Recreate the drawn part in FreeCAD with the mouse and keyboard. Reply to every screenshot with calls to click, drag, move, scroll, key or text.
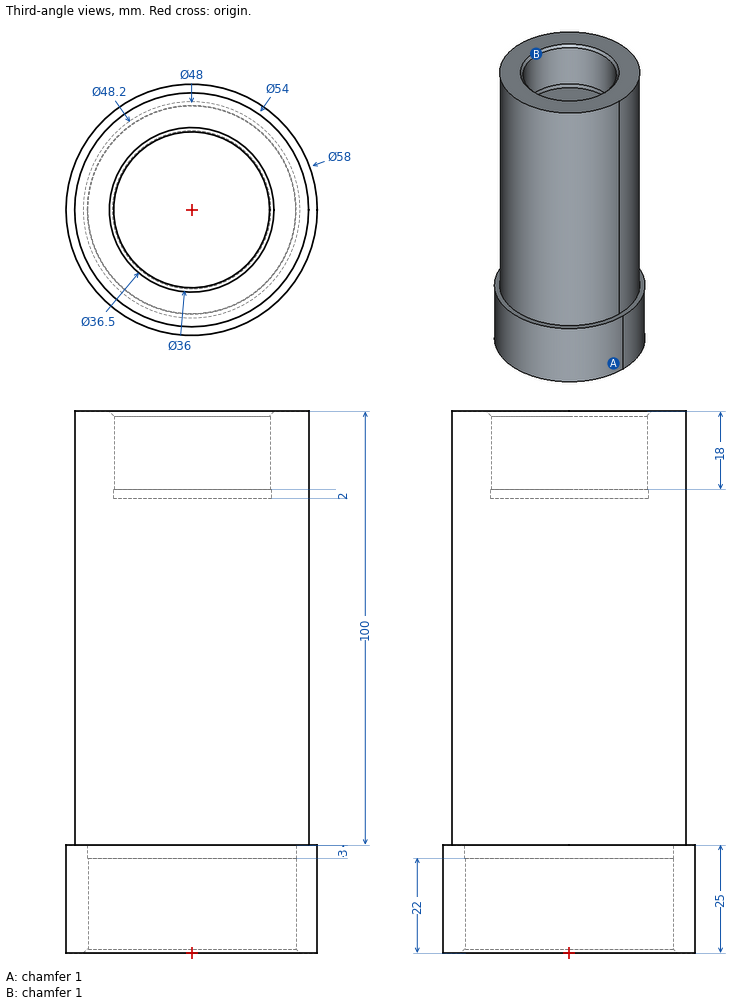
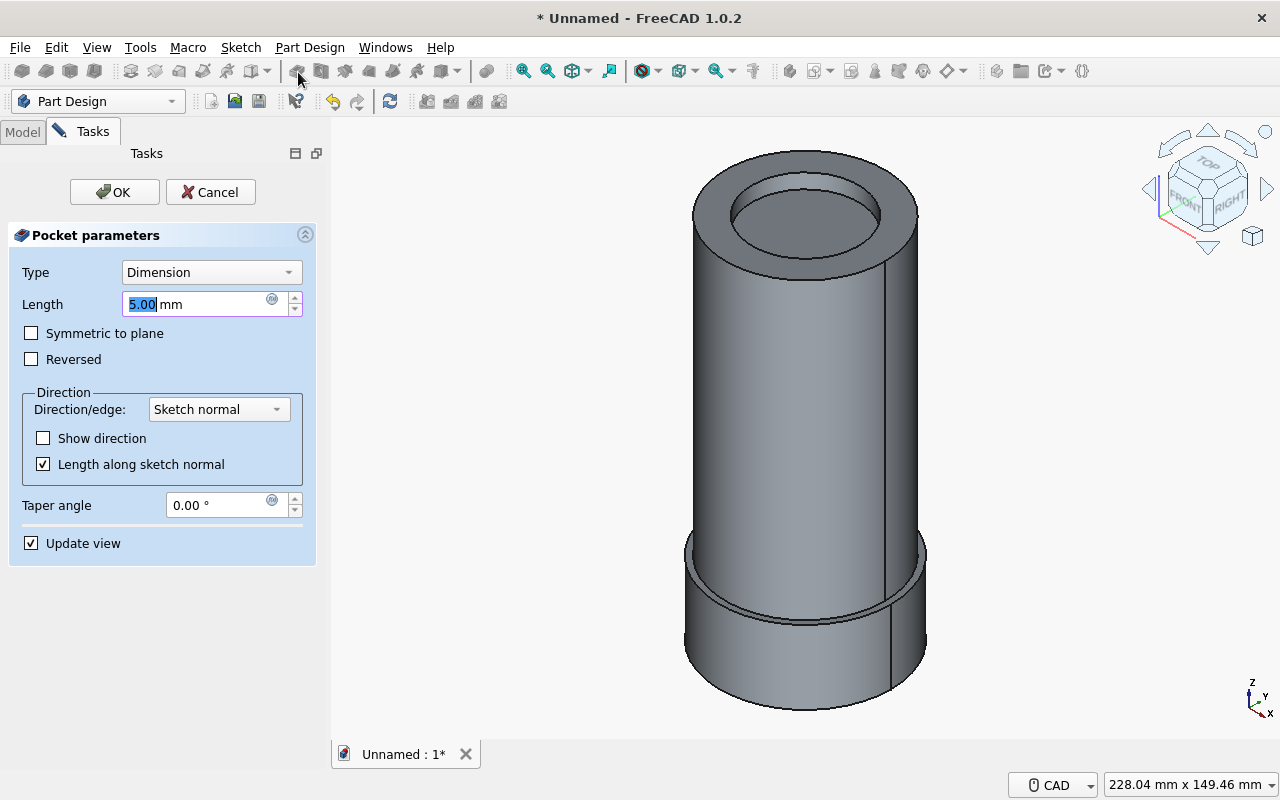
text(18)
key(Tab)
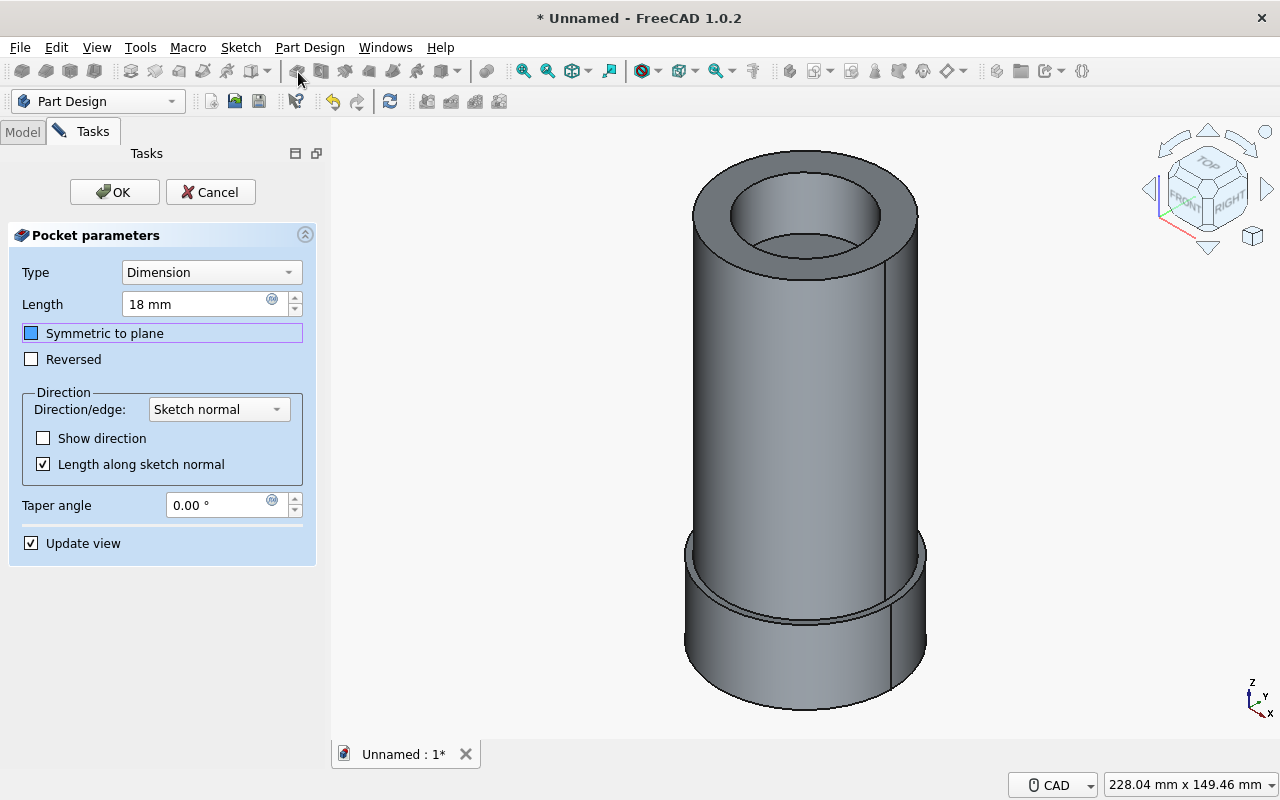
click(115, 192)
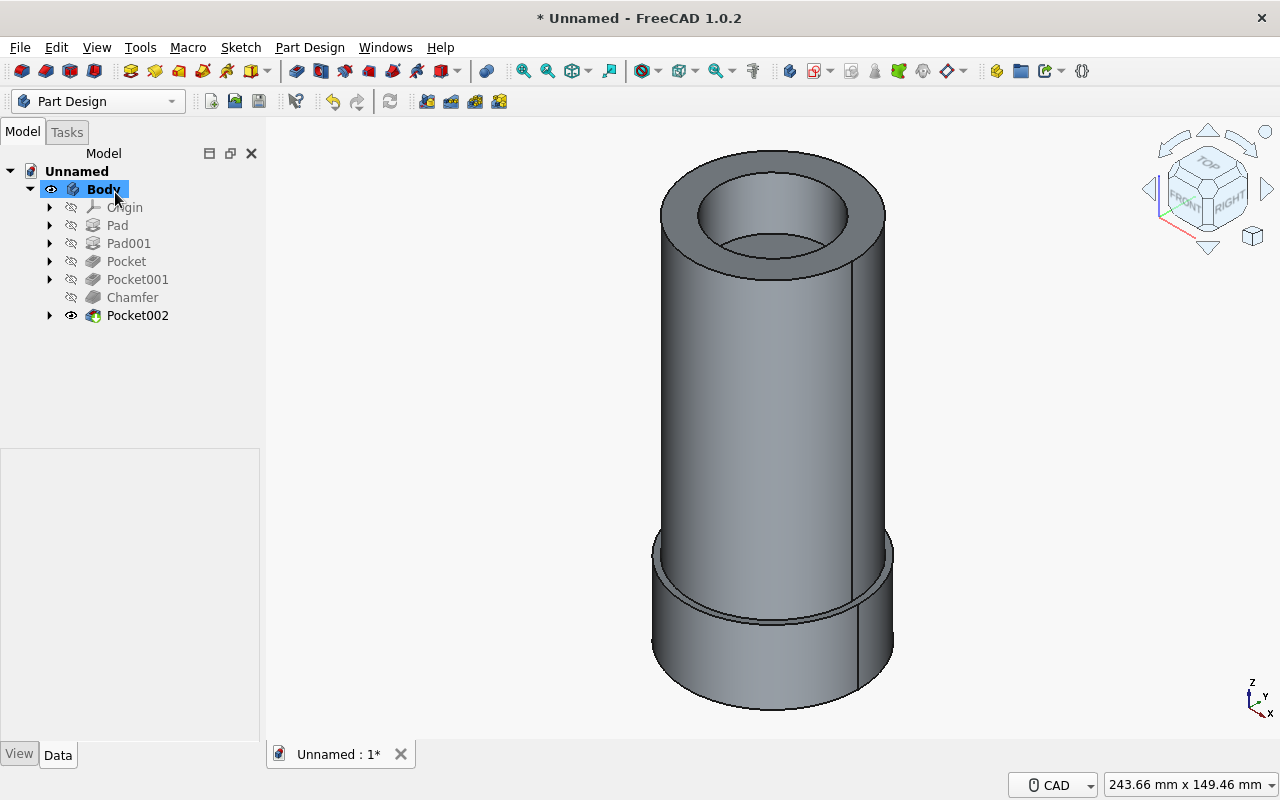
click(524, 72)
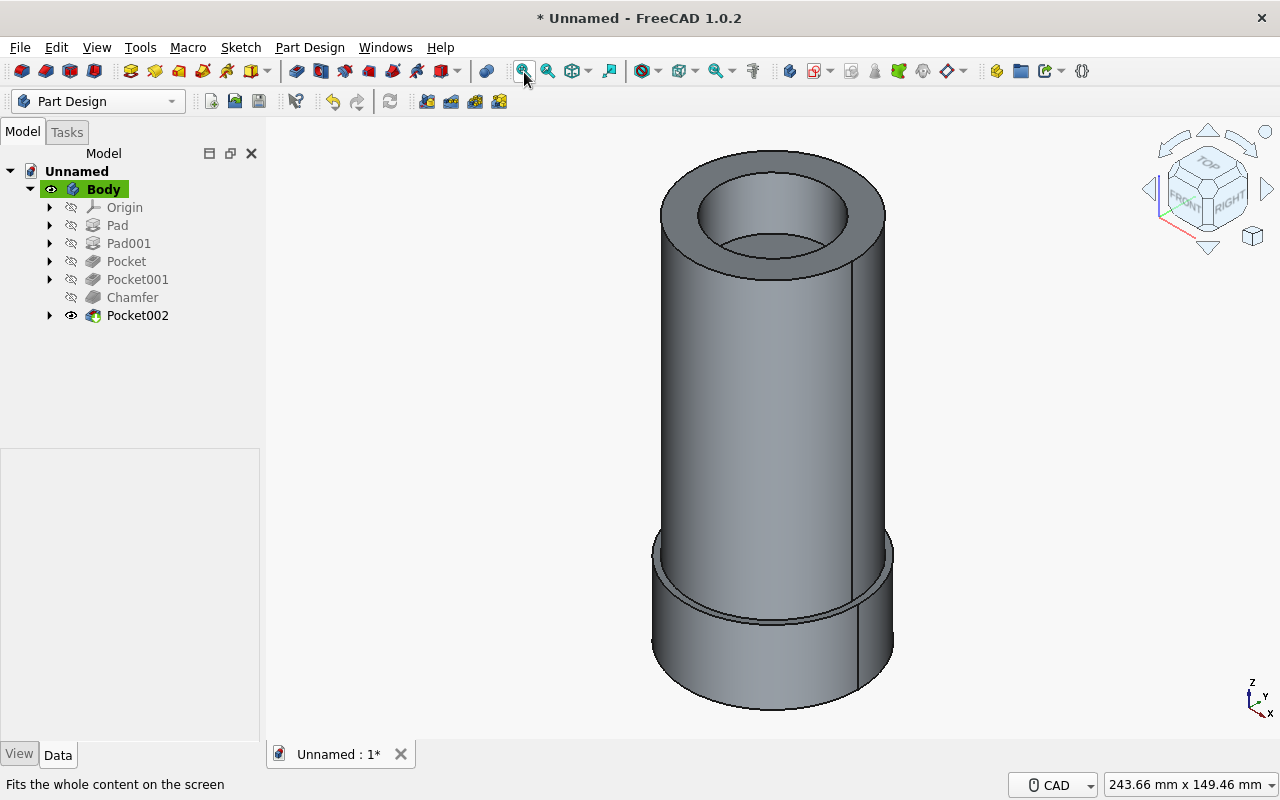
key(2)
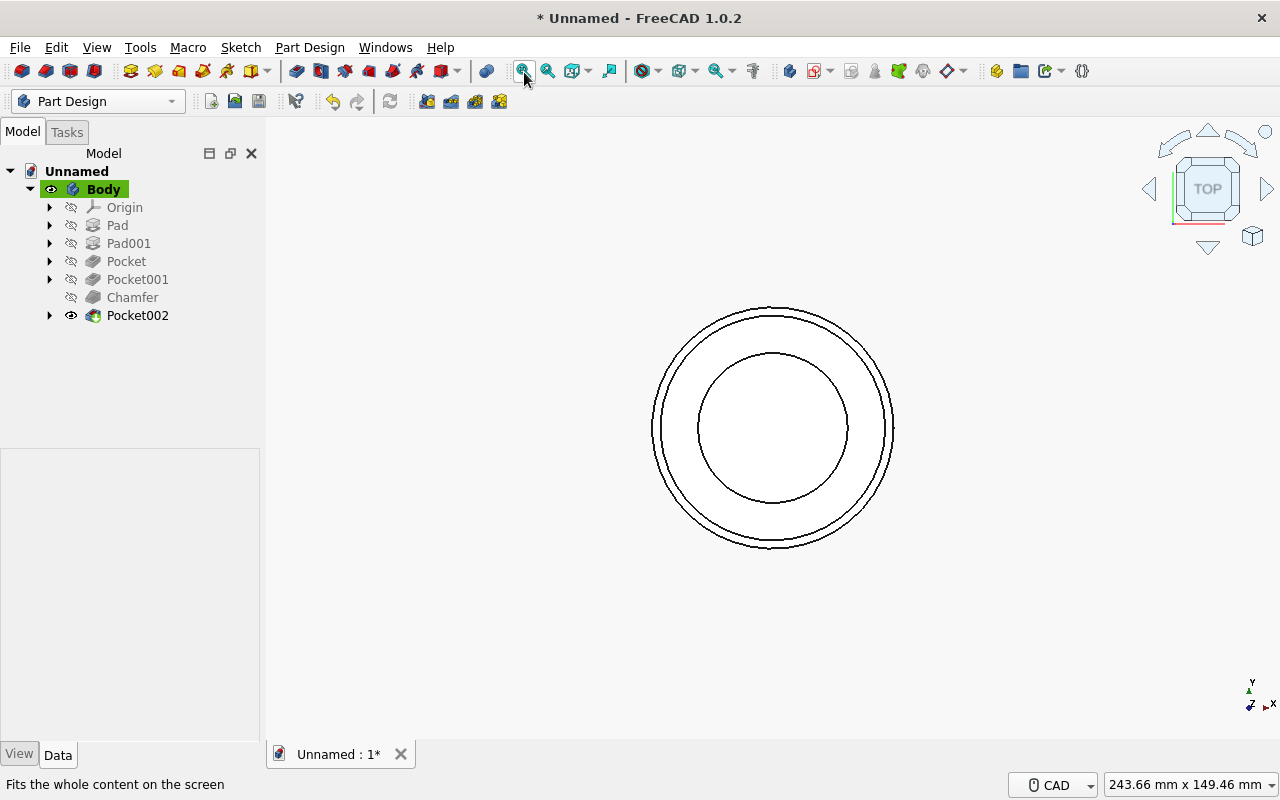
click(524, 72)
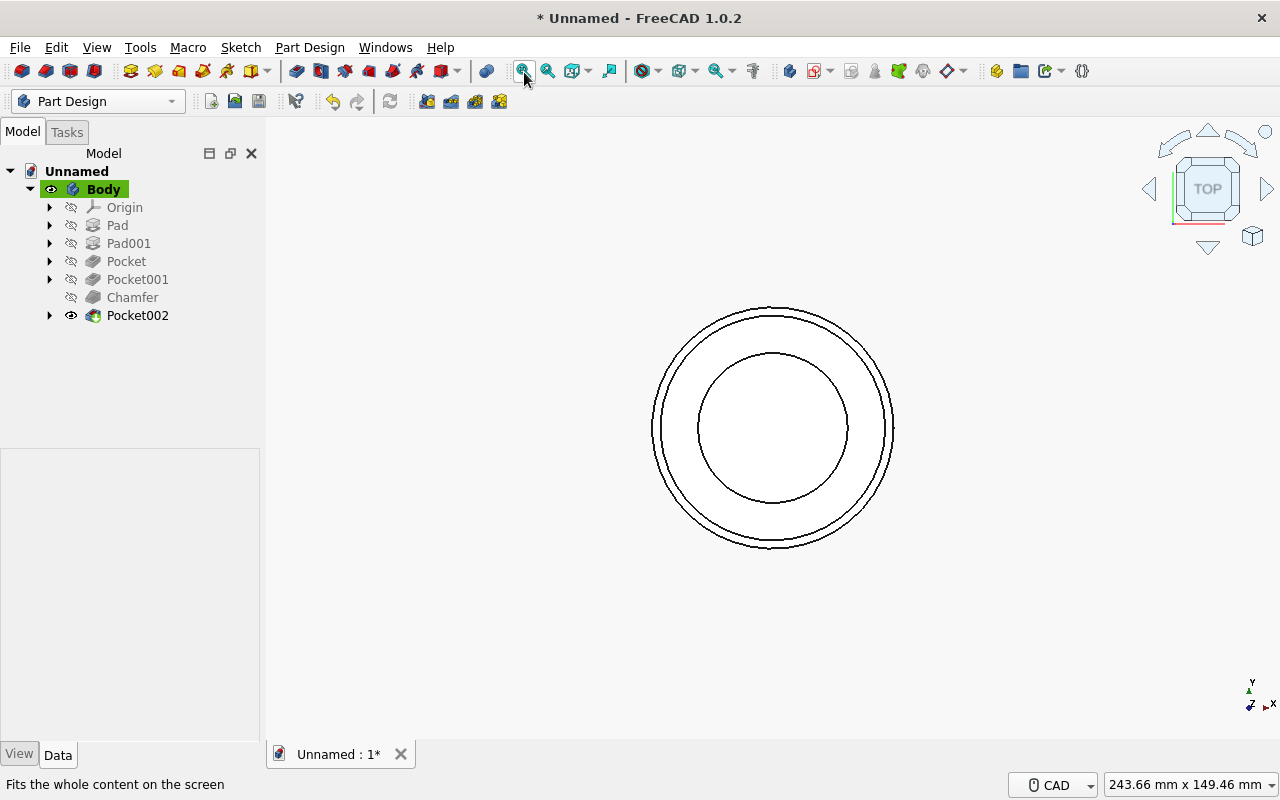
click(773, 427)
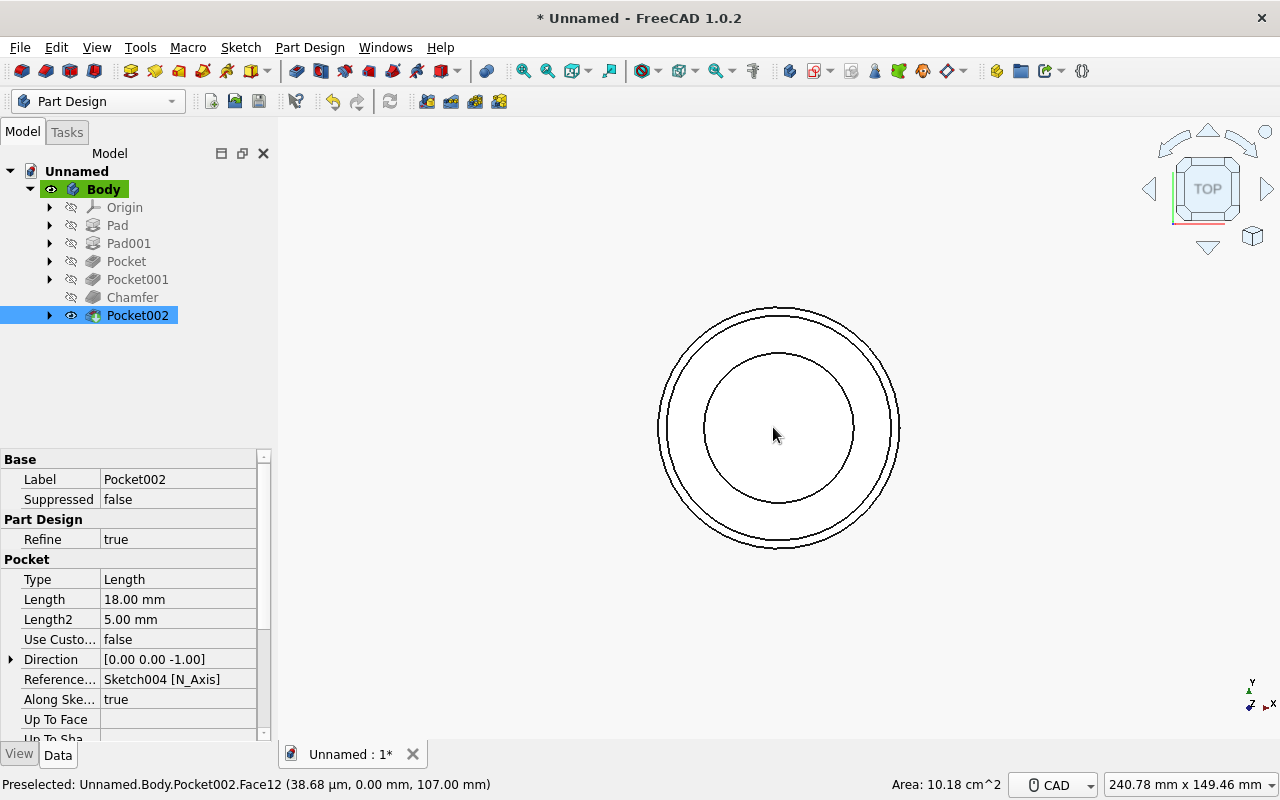
click(814, 72)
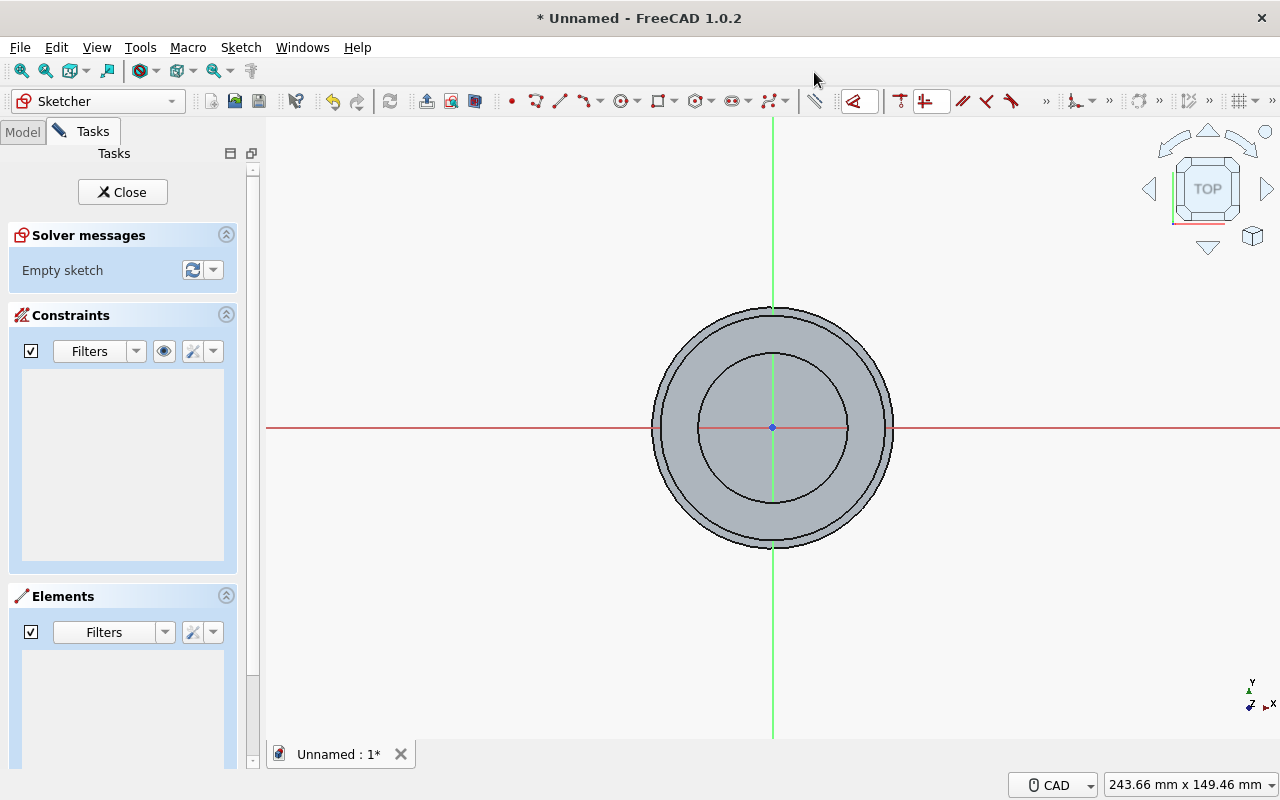
scroll(813, 428, up, 5)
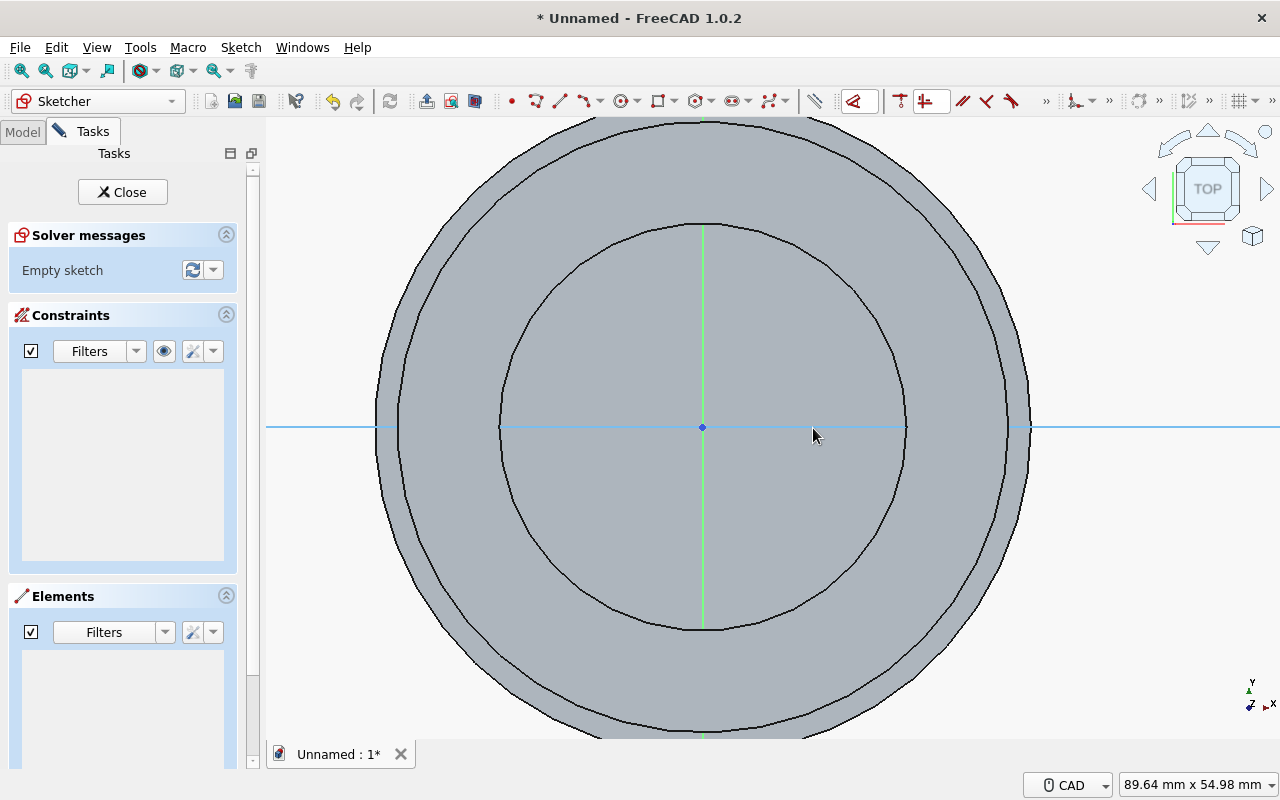
click(622, 102)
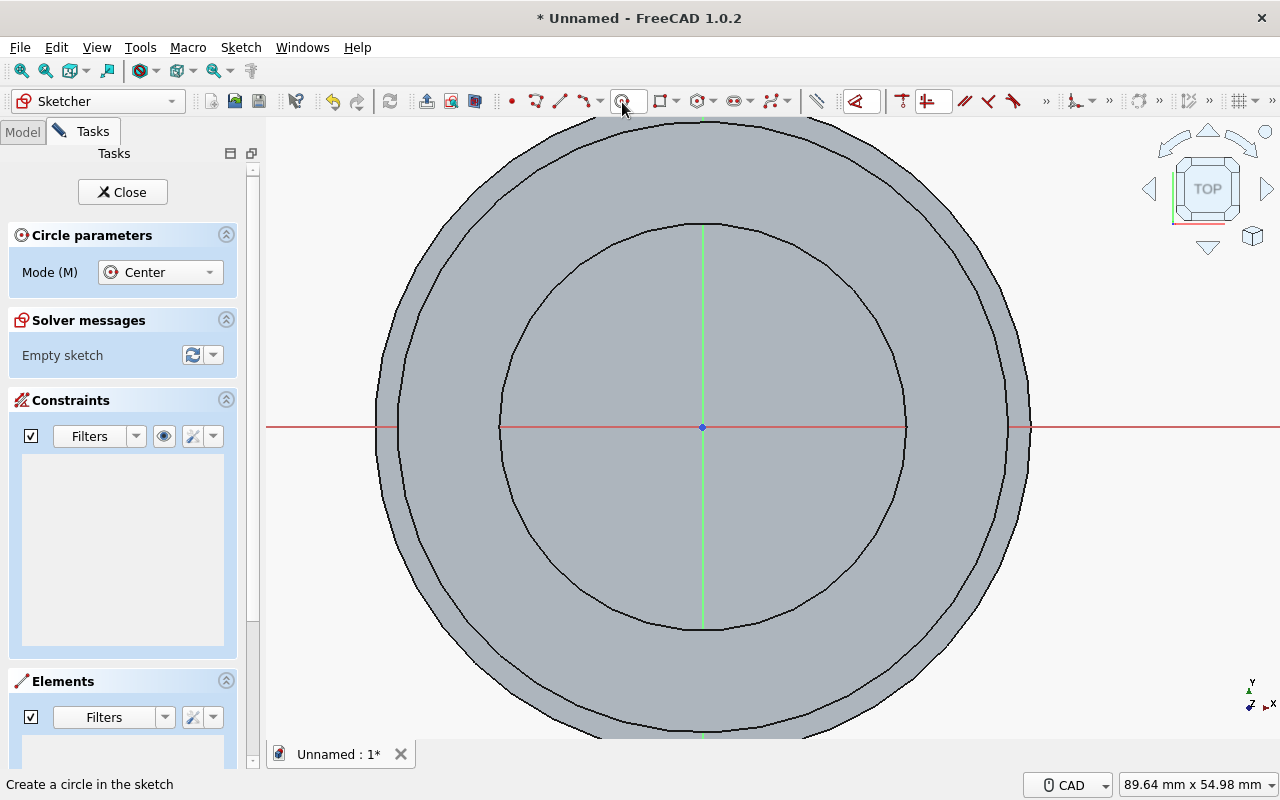
click(703, 427)
move(849, 281)